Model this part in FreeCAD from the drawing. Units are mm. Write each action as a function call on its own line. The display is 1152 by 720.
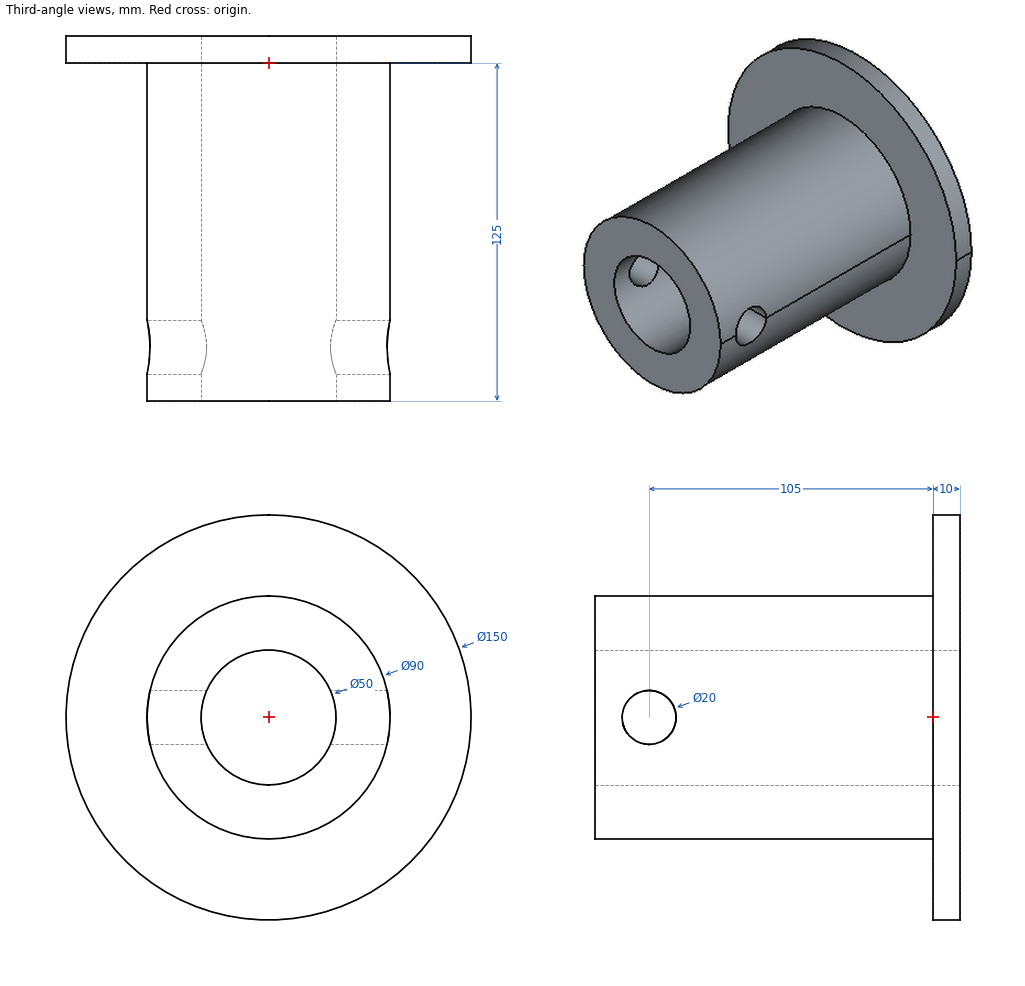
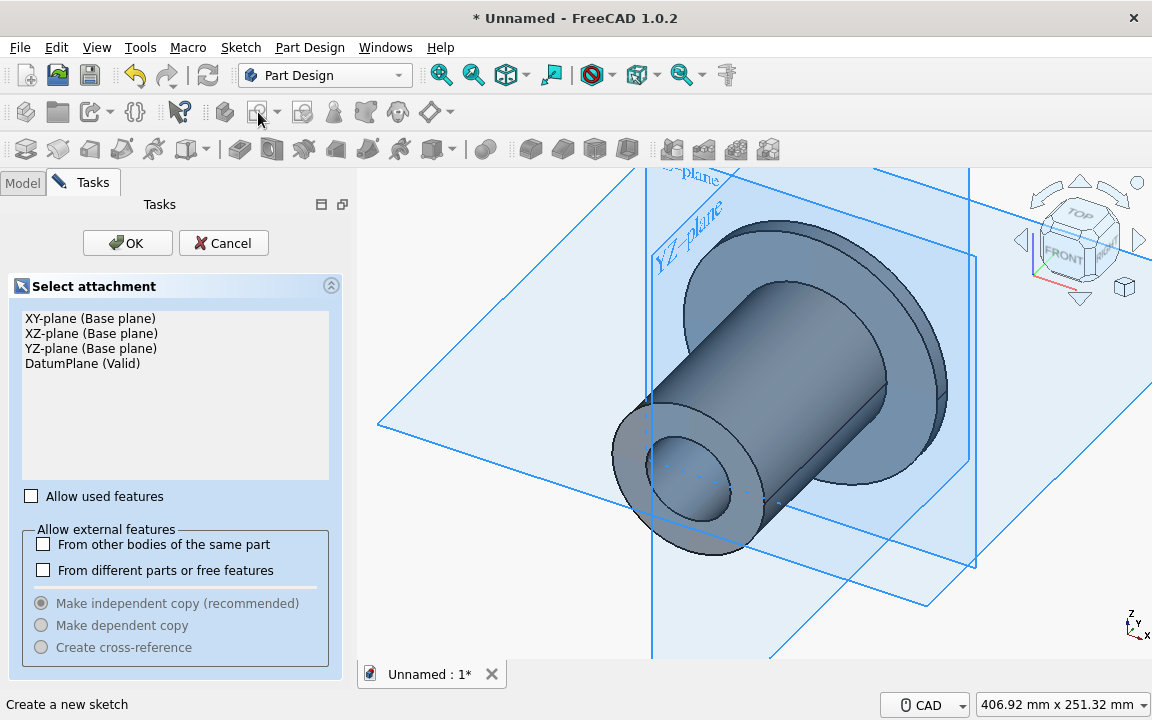
click(82, 348)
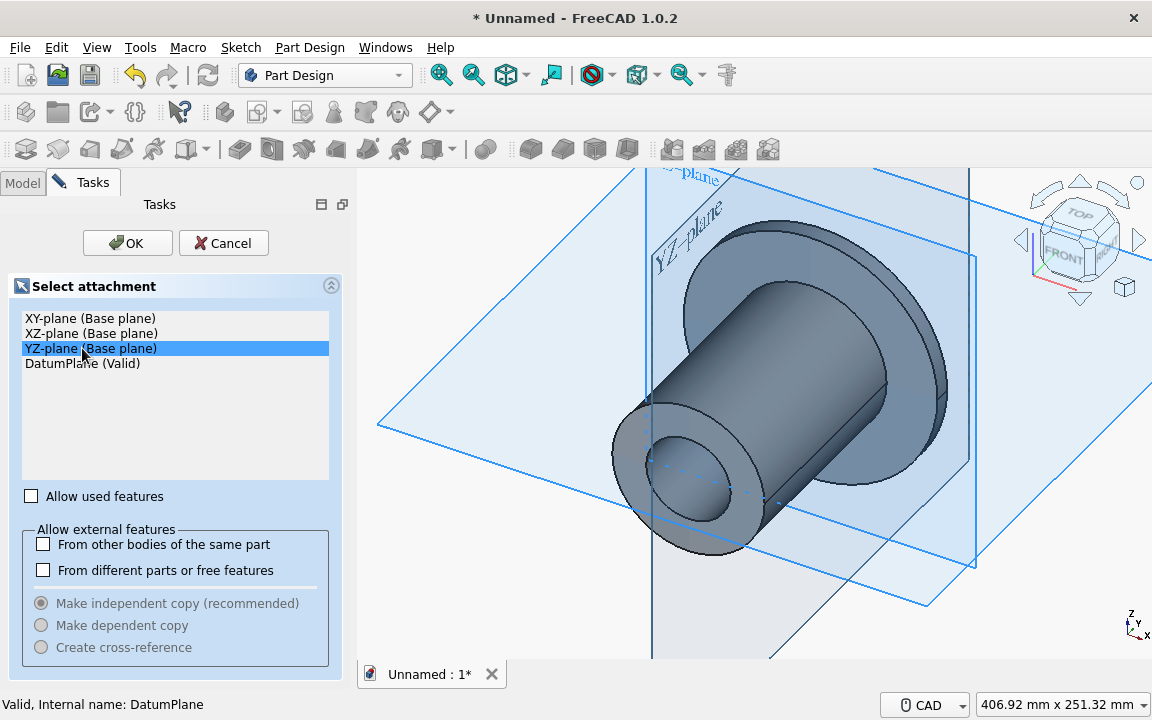
click(128, 243)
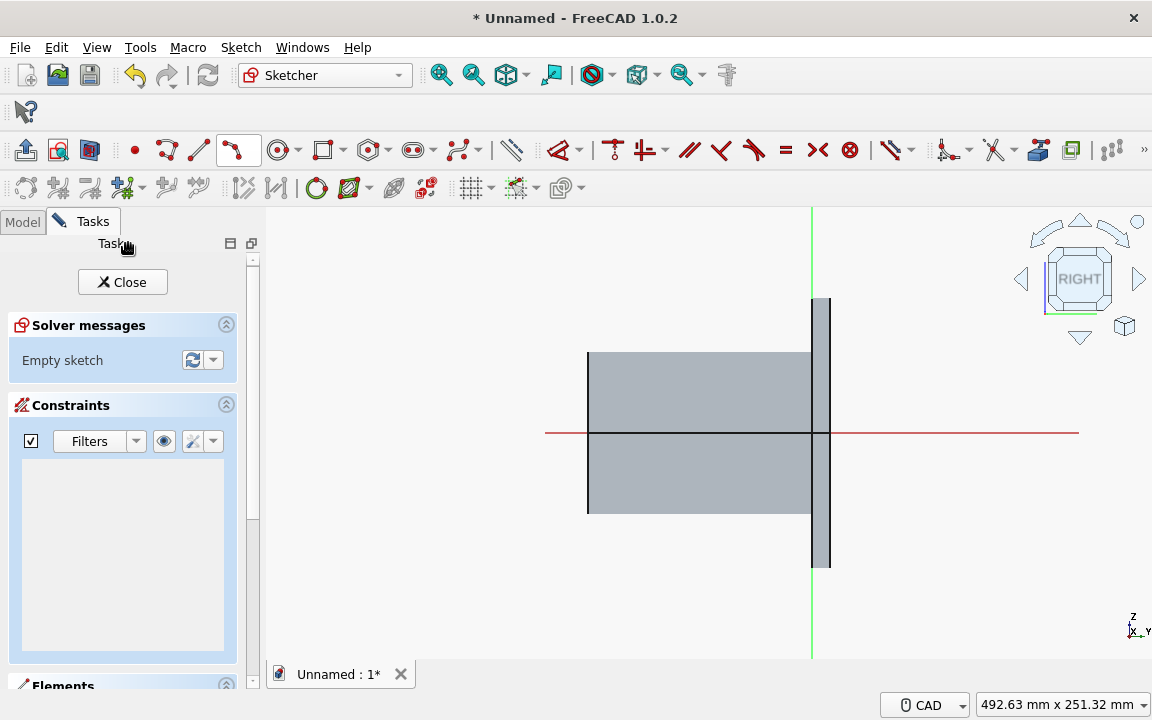
click(90, 150)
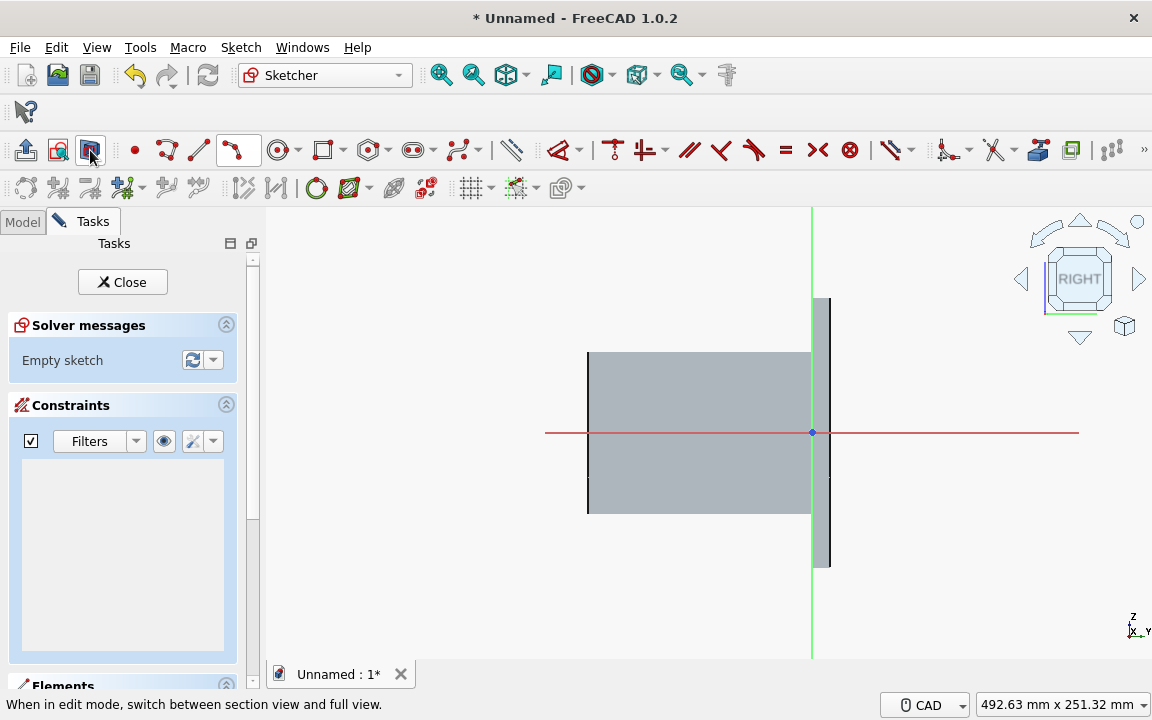
scroll(621, 433, up, 10)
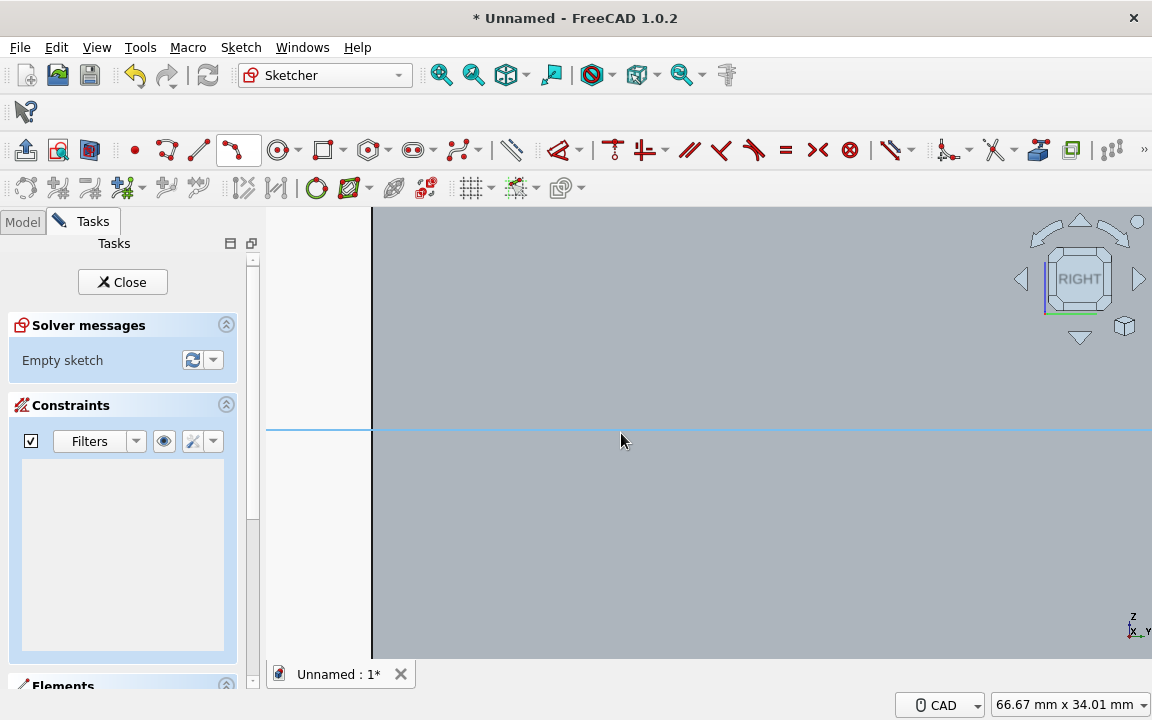
click(278, 150)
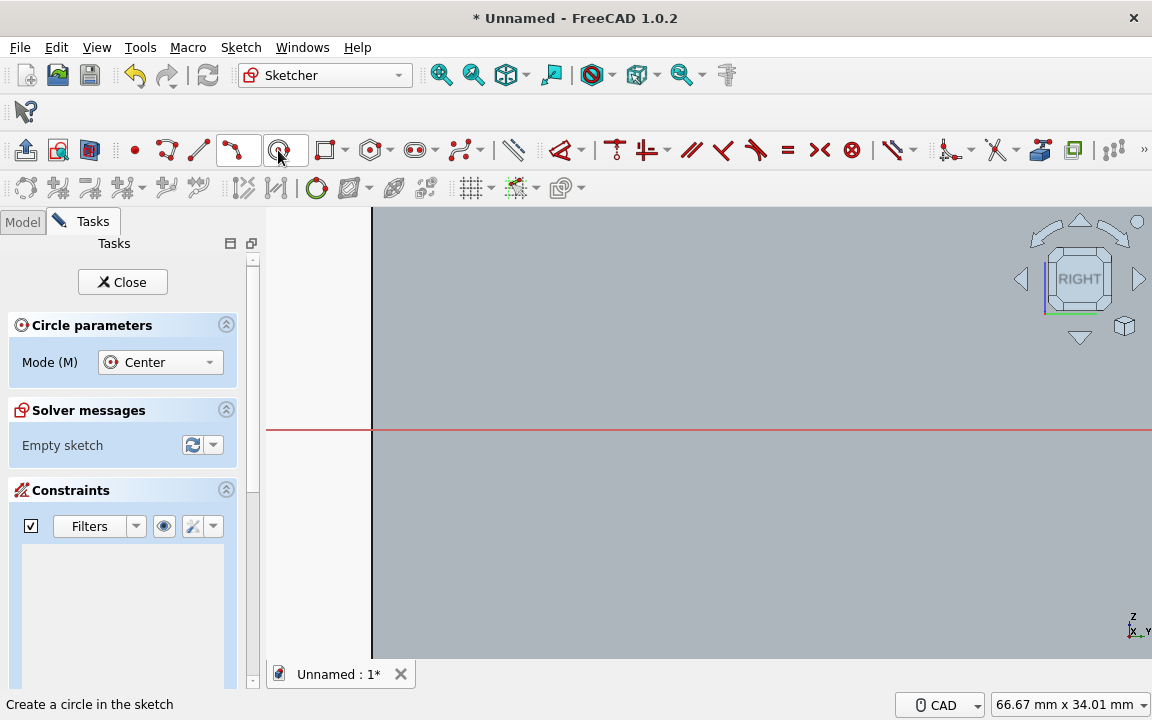
click(637, 430)
click(731, 336)
key(Escape)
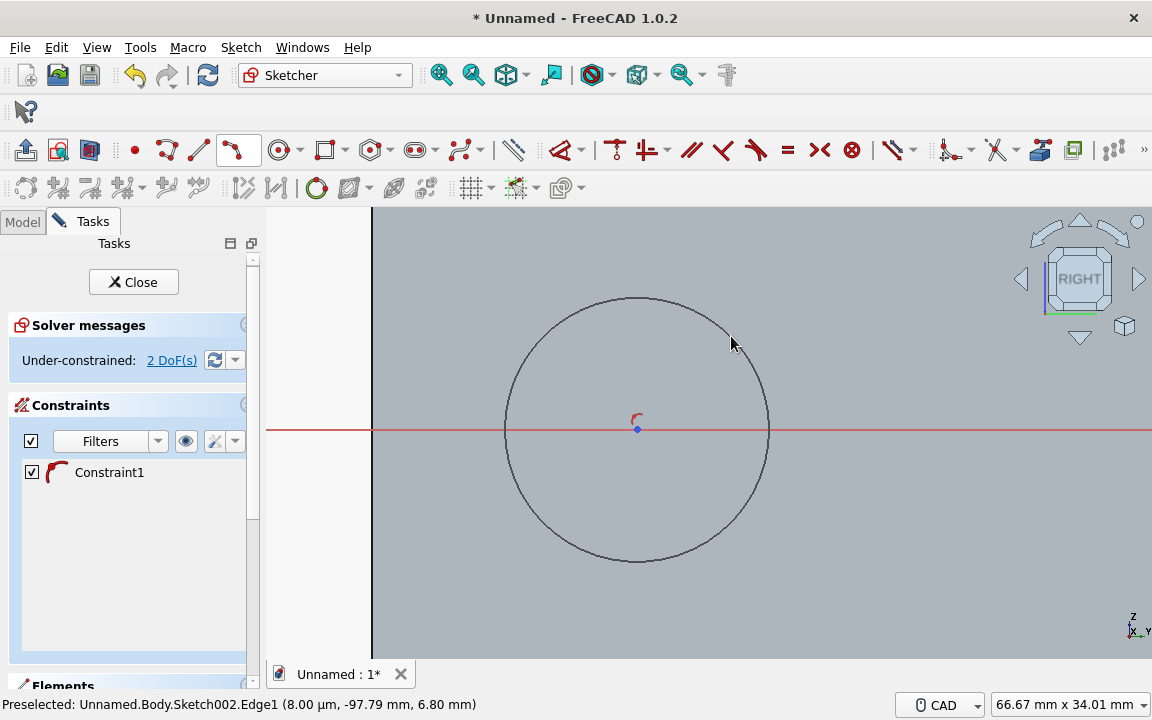
click(560, 150)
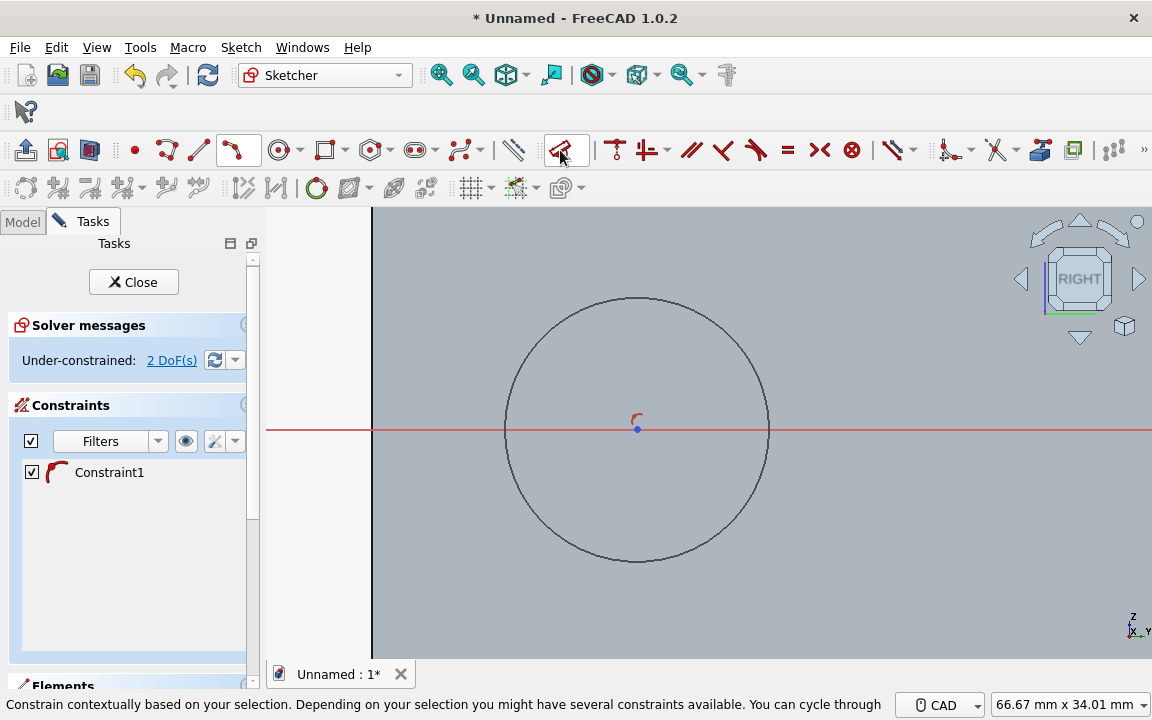
click(730, 336)
click(753, 313)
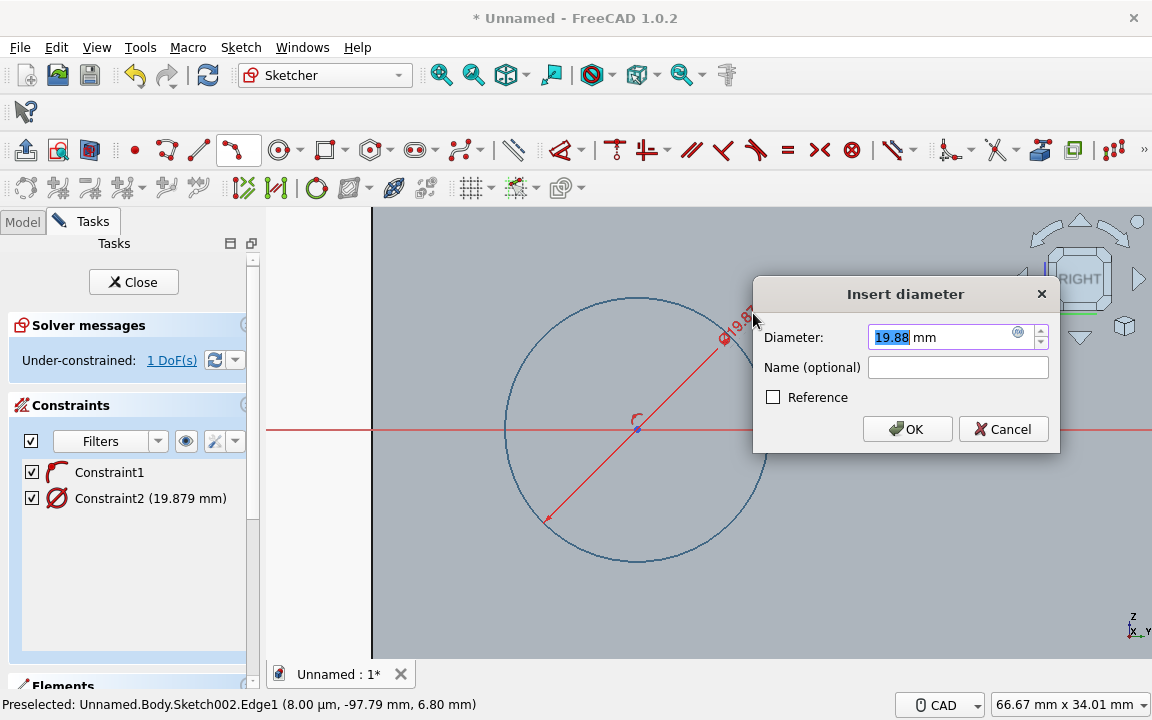
text(20)
key(Return)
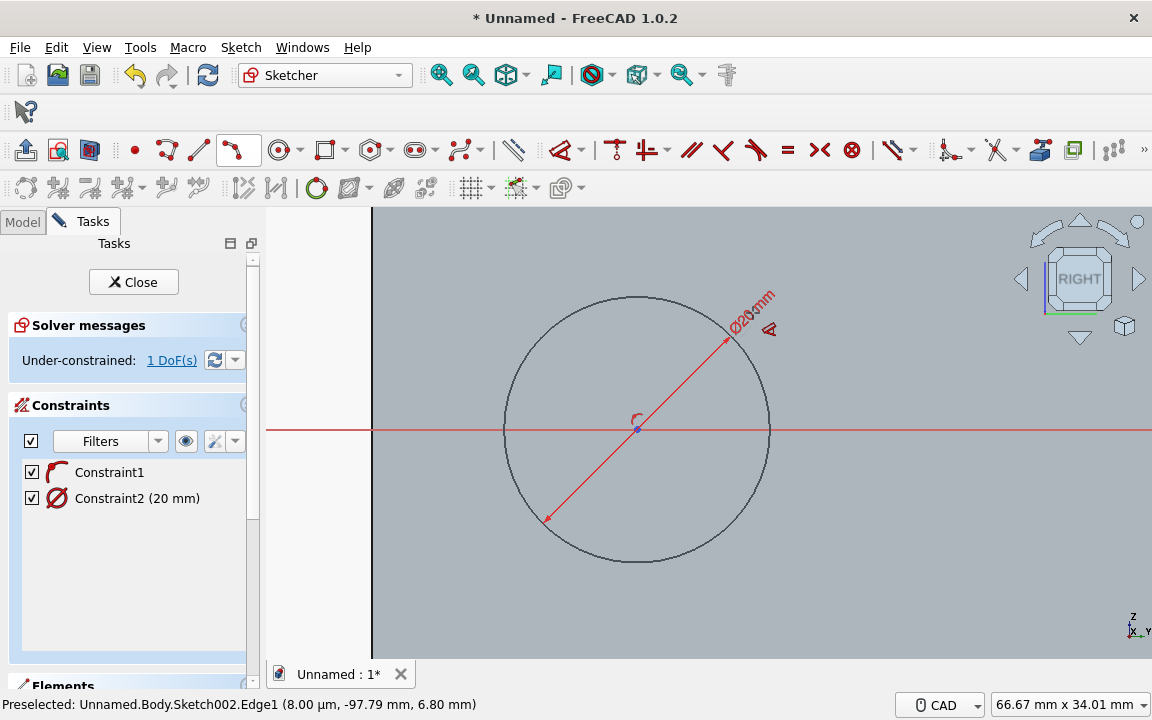
click(637, 430)
click(812, 464)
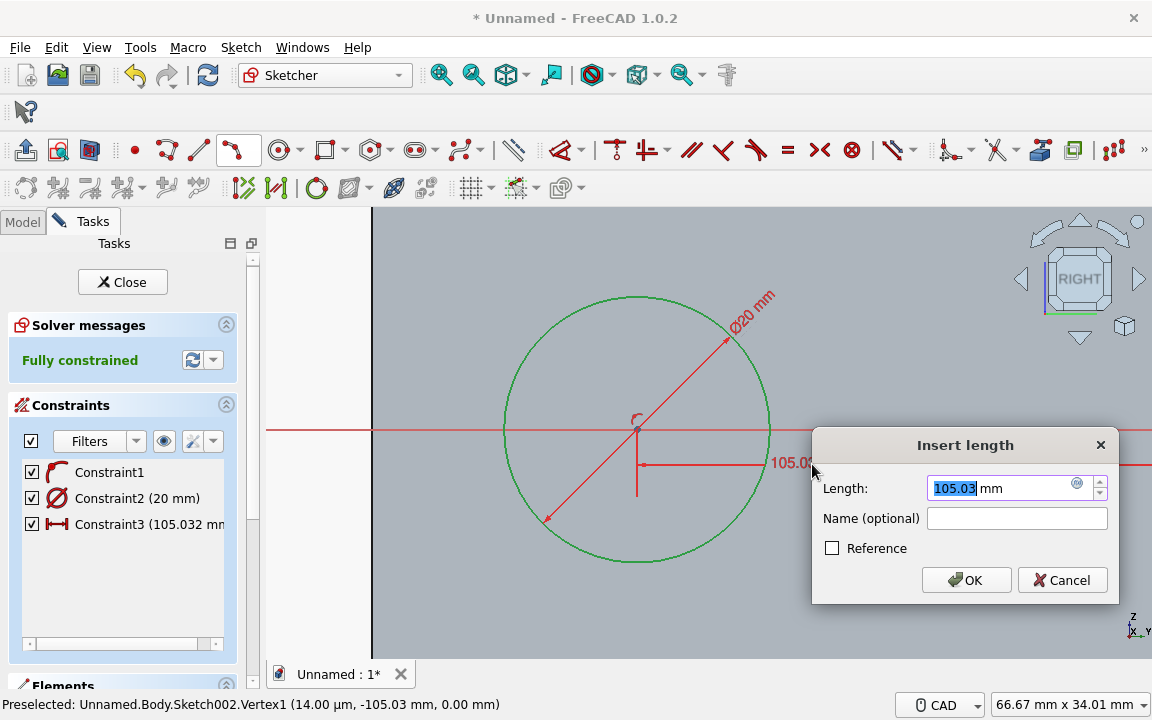
text(105)
key(Return)
key(Escape)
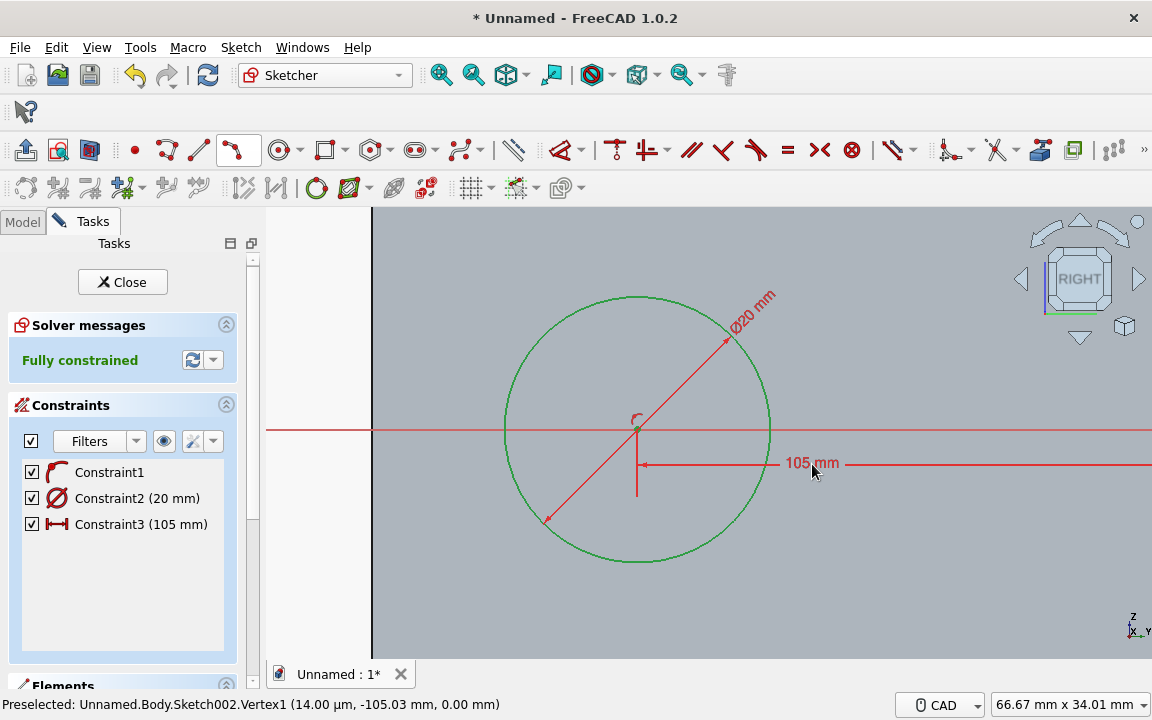
click(123, 282)